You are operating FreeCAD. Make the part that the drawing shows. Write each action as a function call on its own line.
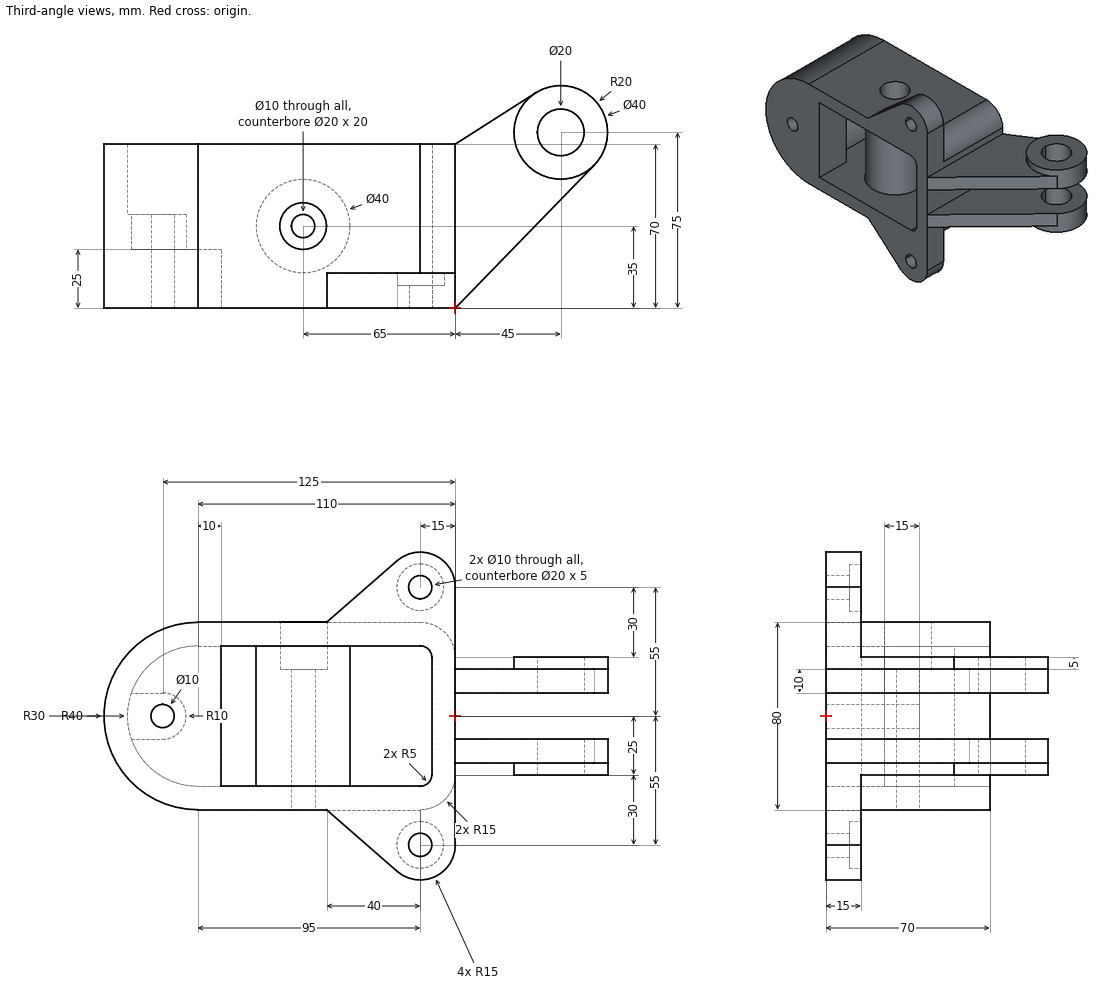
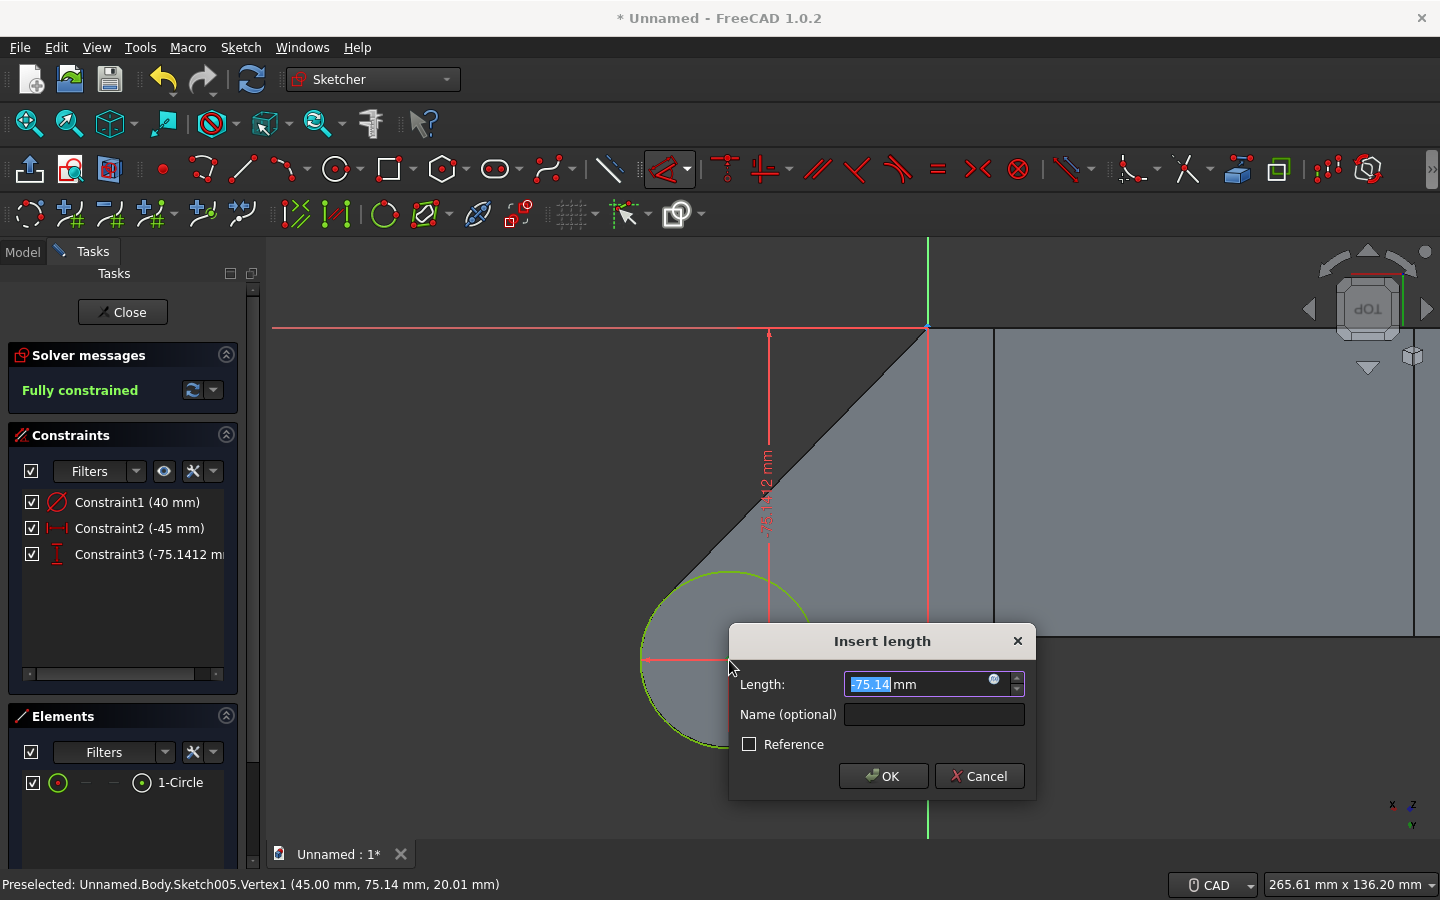
text(-75)
key(Return)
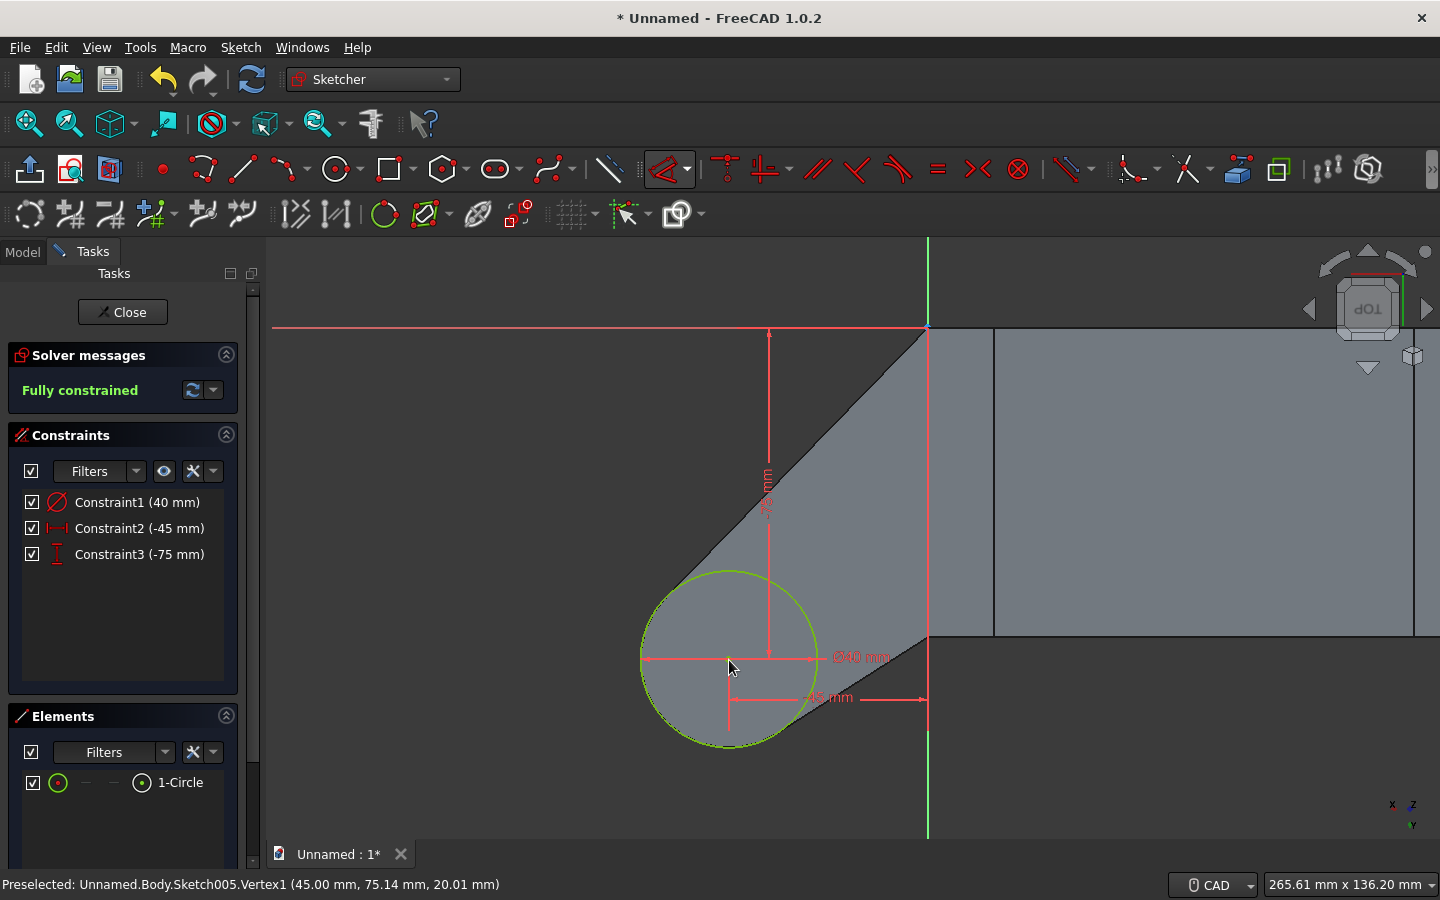
click(123, 312)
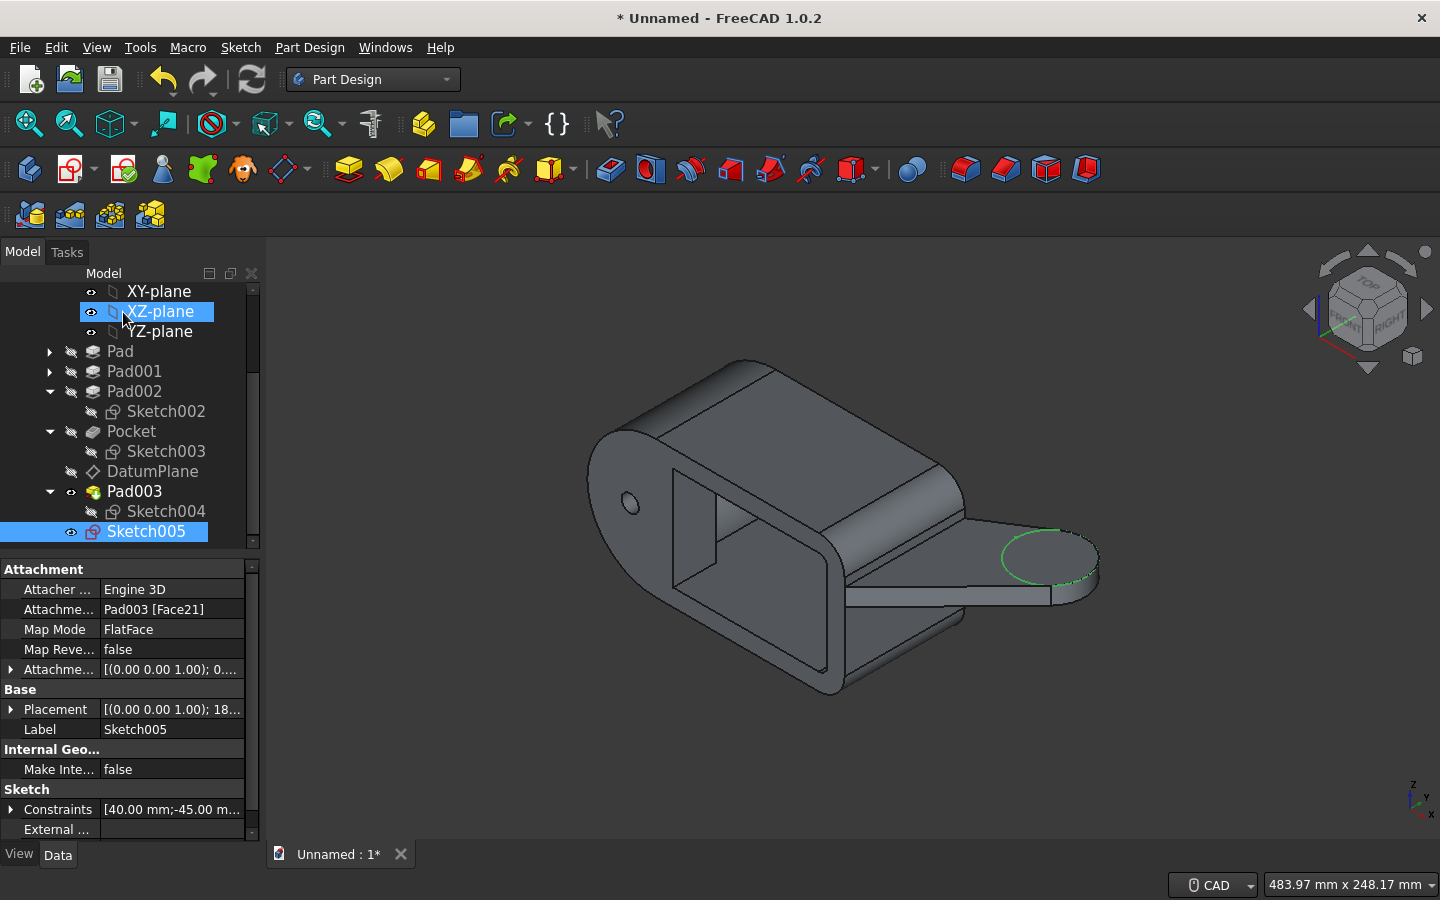
click(350, 170)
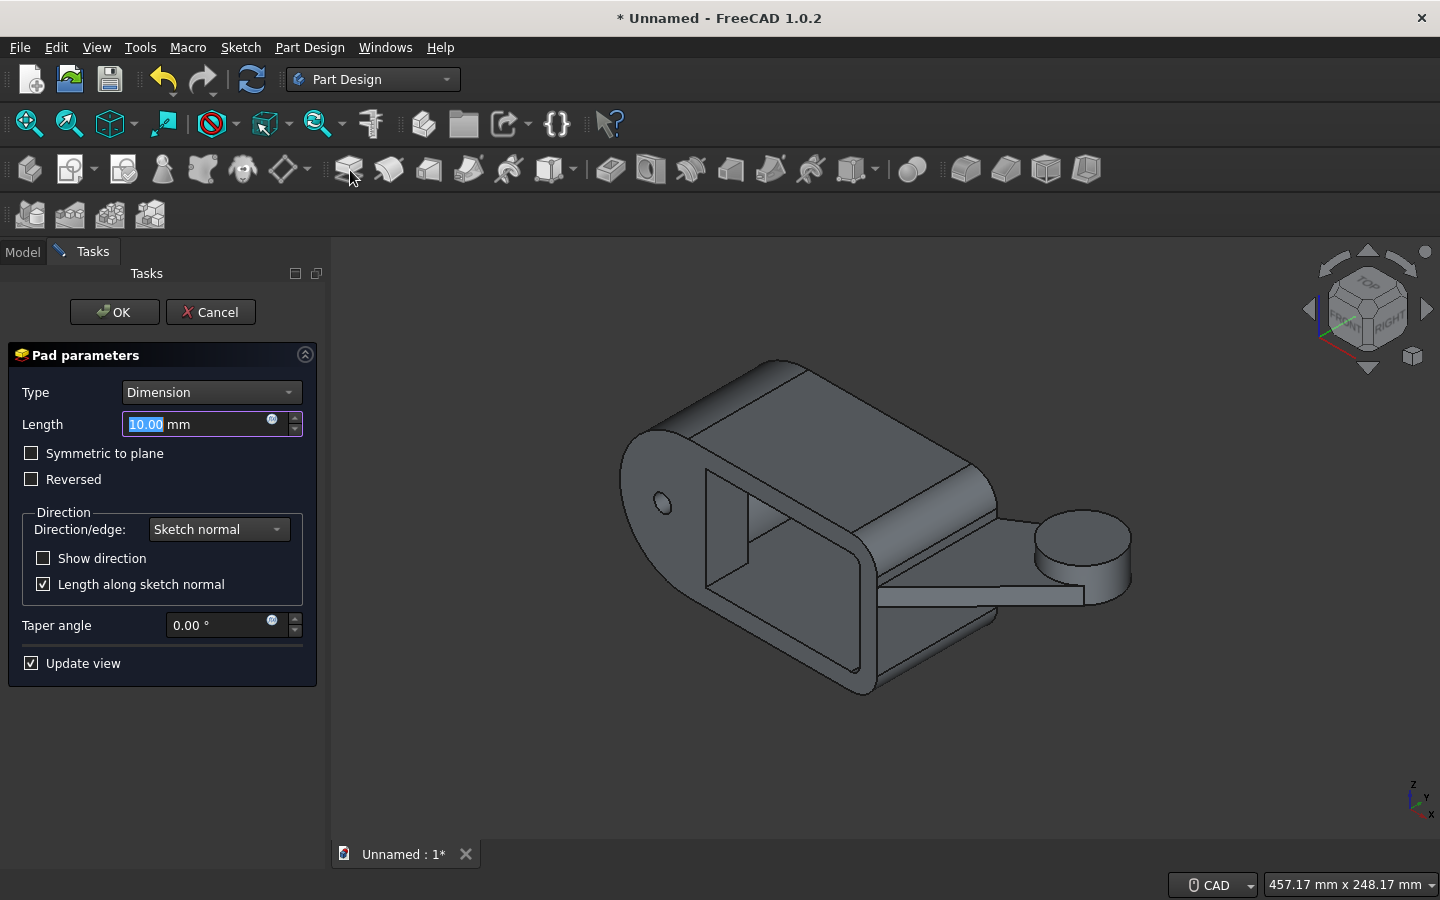
text(5)
key(Tab)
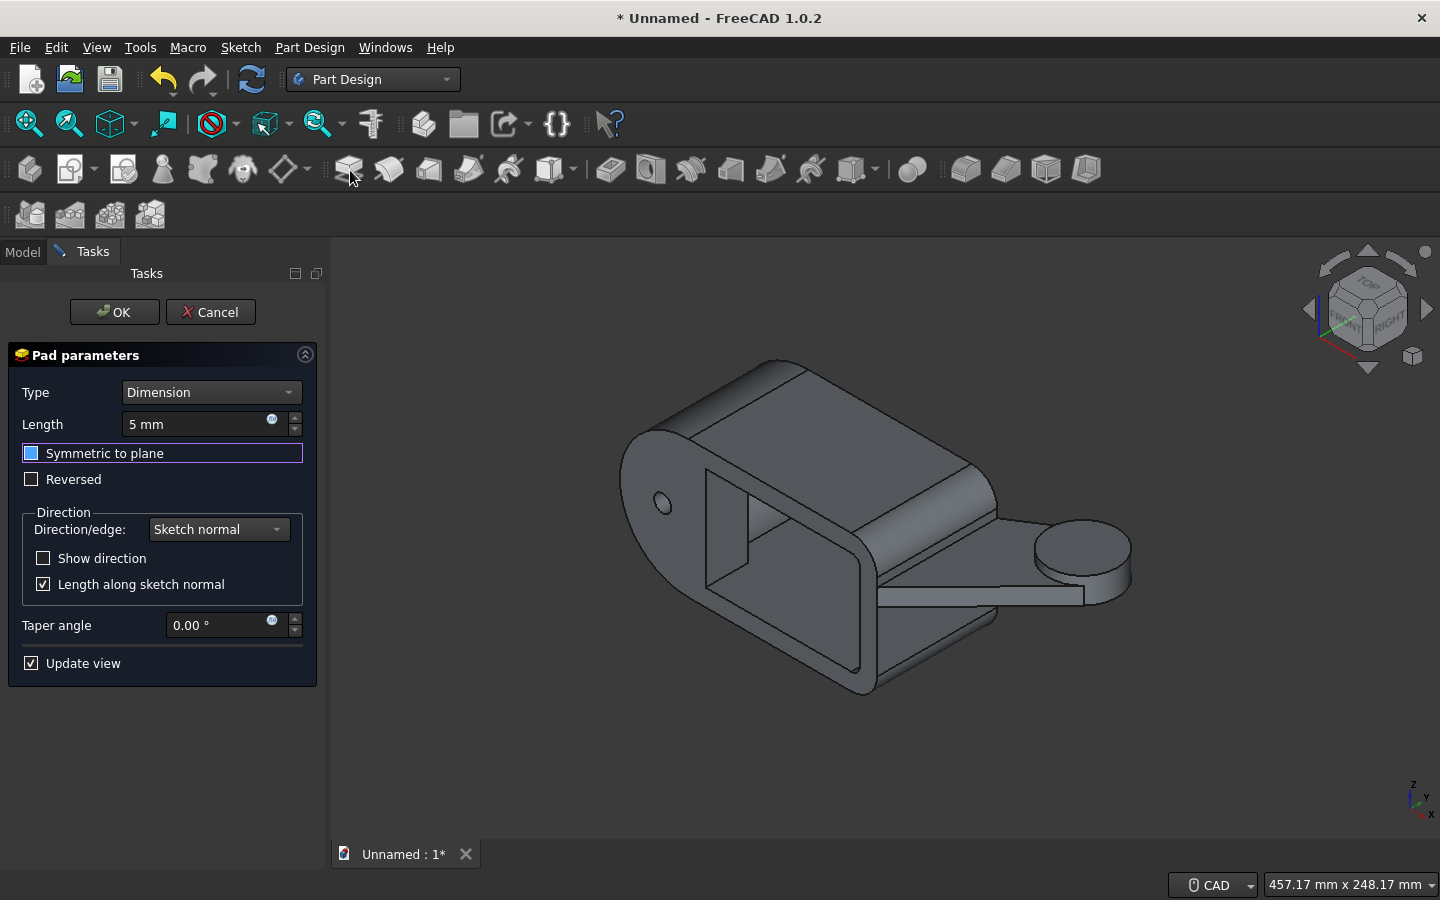
click(115, 312)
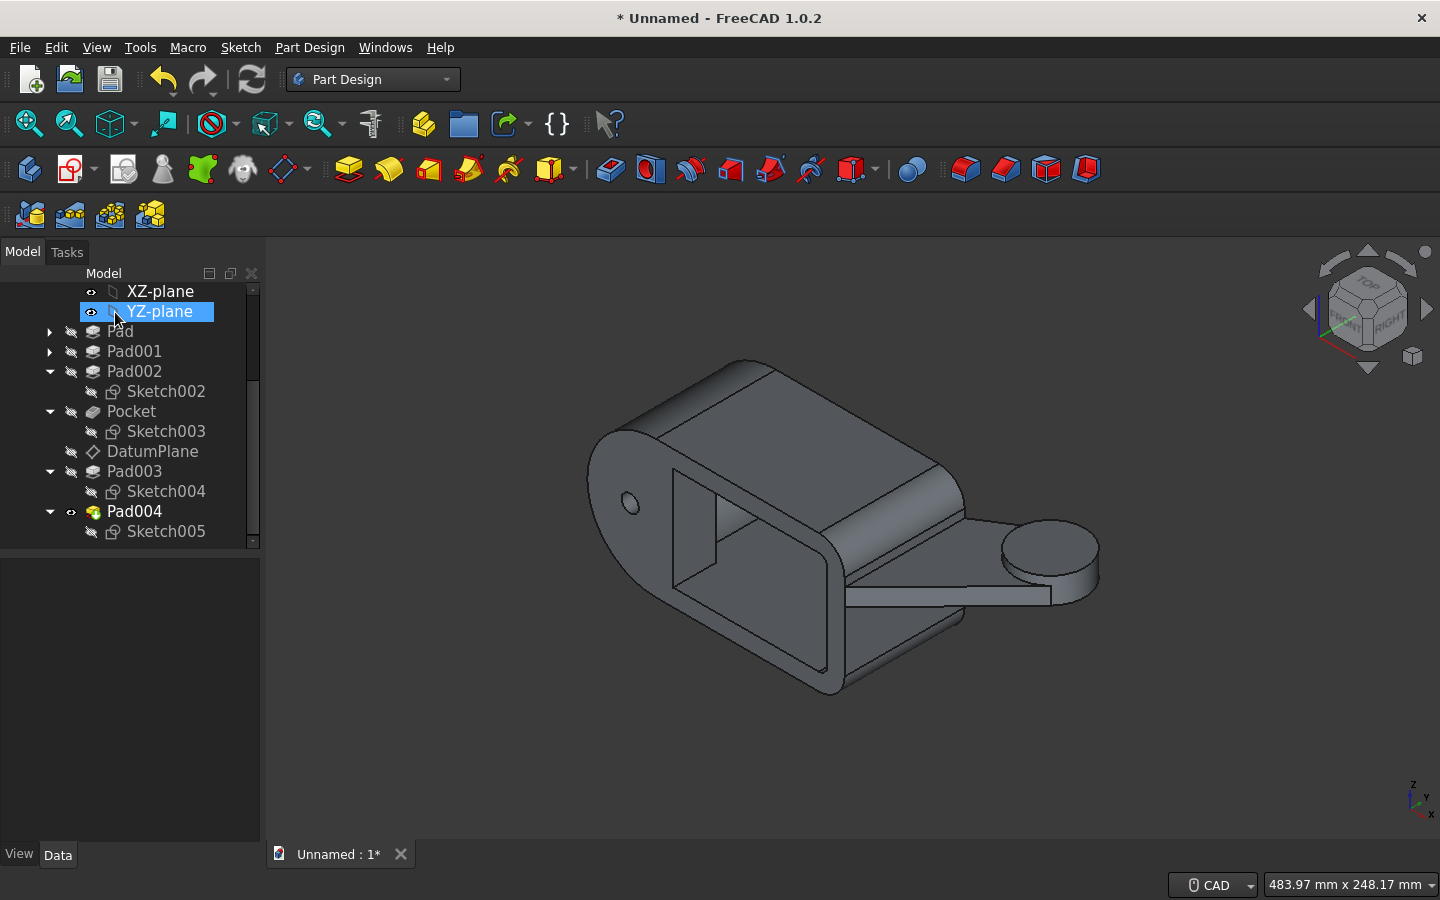
click(116, 472)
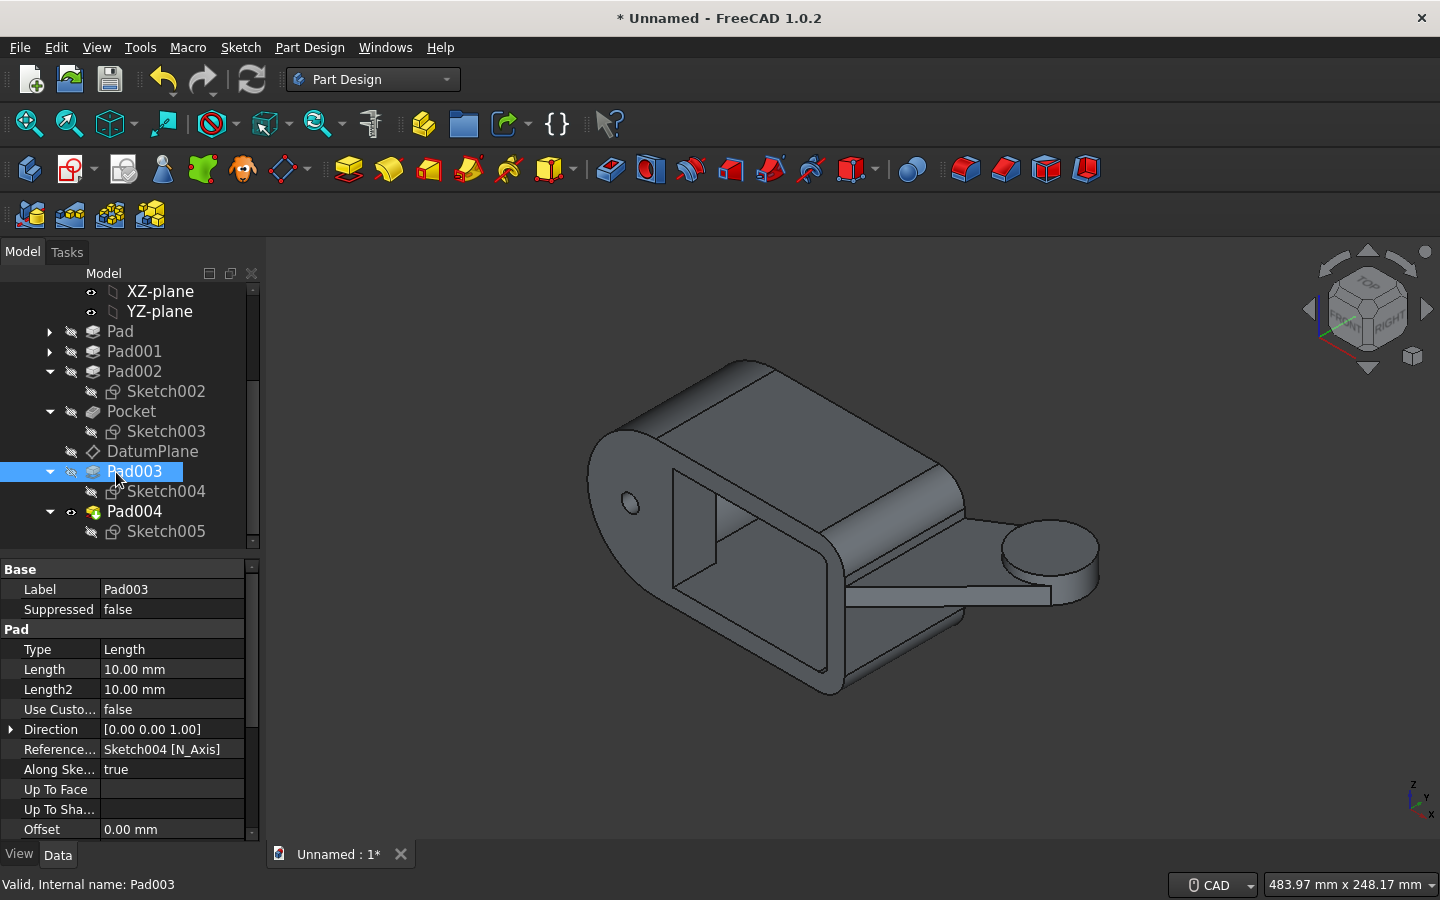
click(116, 512, ctrl)